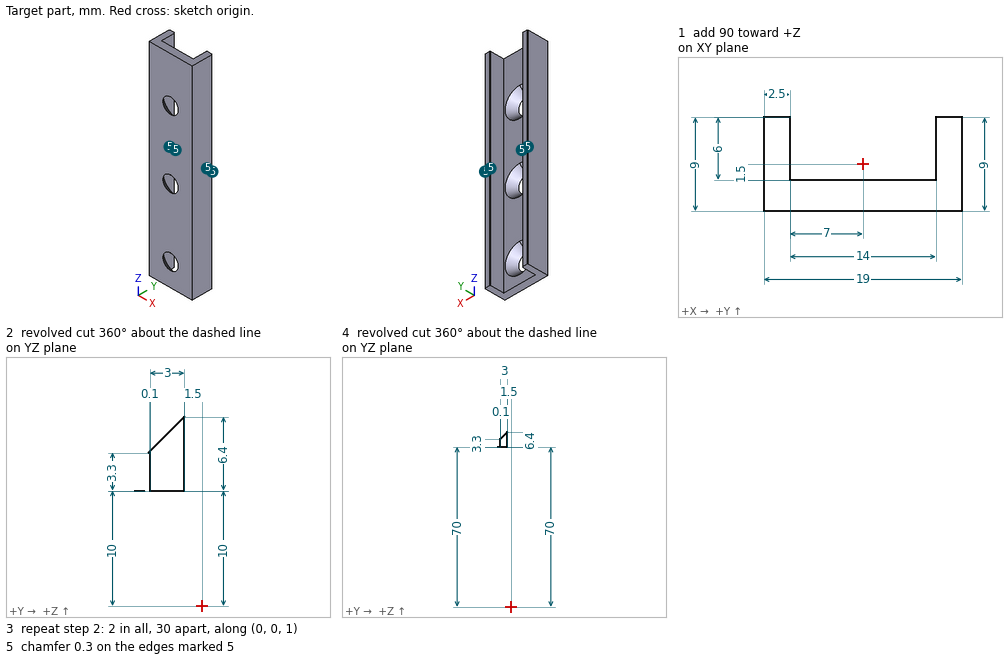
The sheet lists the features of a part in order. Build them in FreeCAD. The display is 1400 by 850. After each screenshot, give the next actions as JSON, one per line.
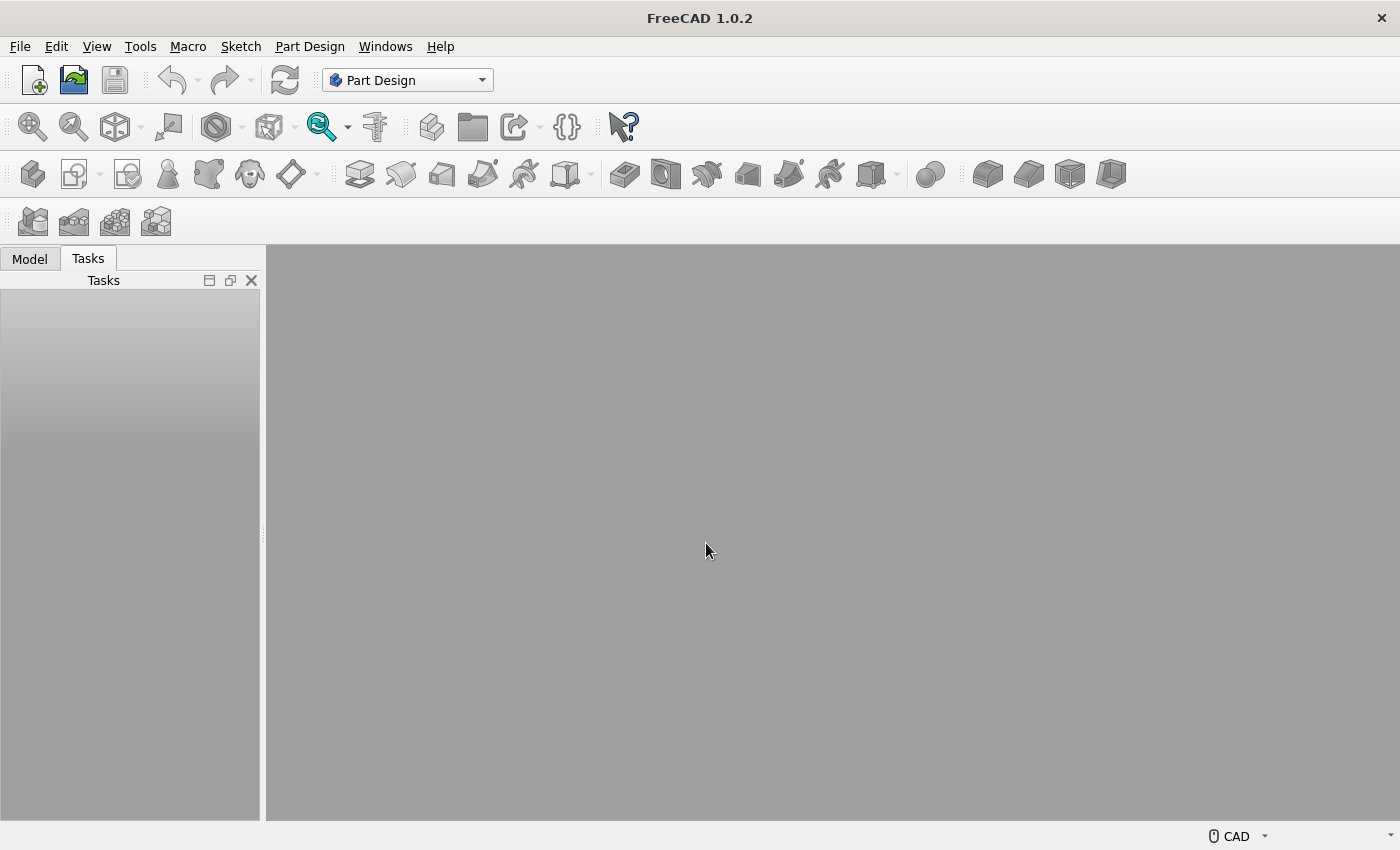
{"action": "left_click", "coordinate": [33, 80]}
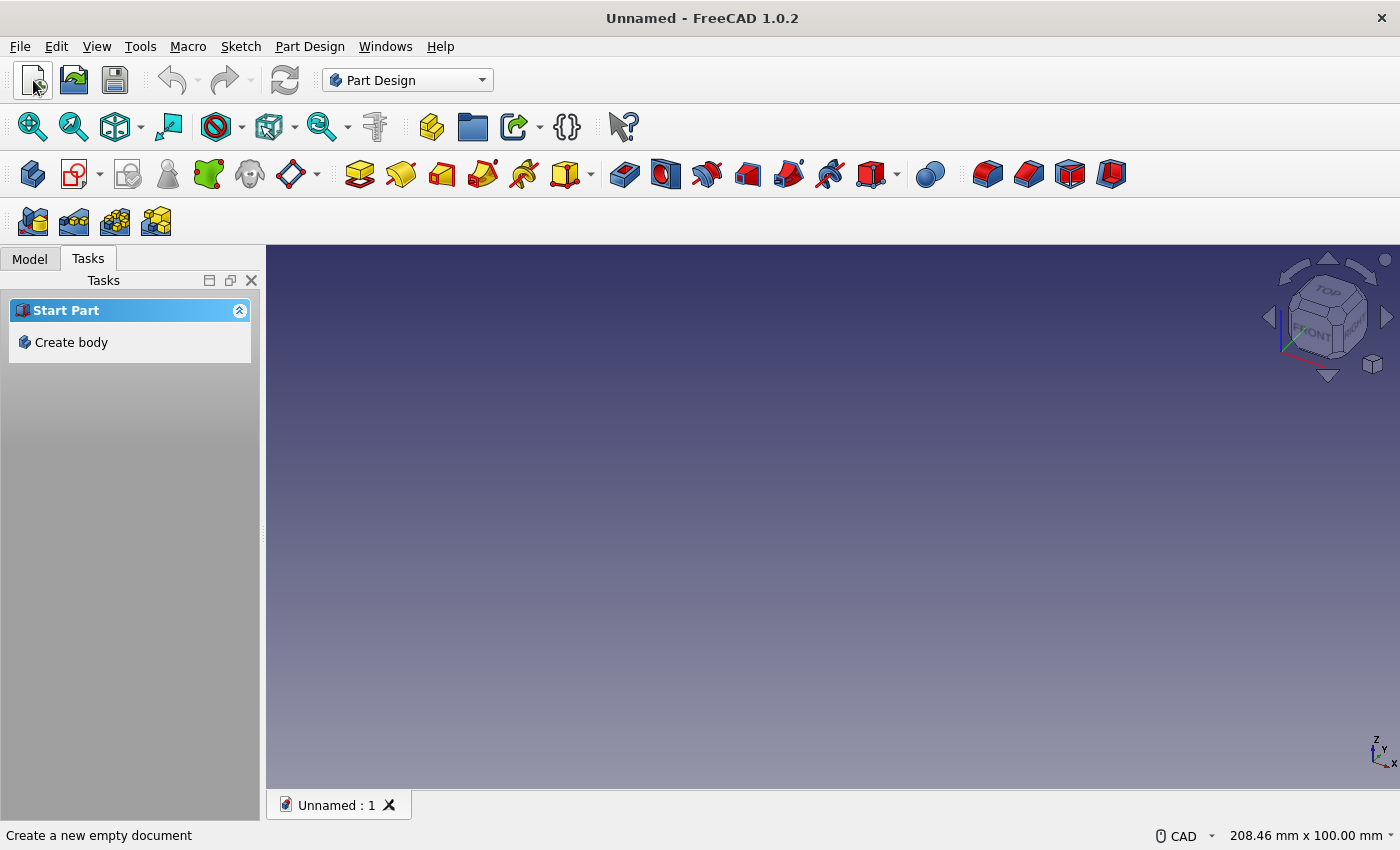
{"action": "left_click", "coordinate": [74, 174]}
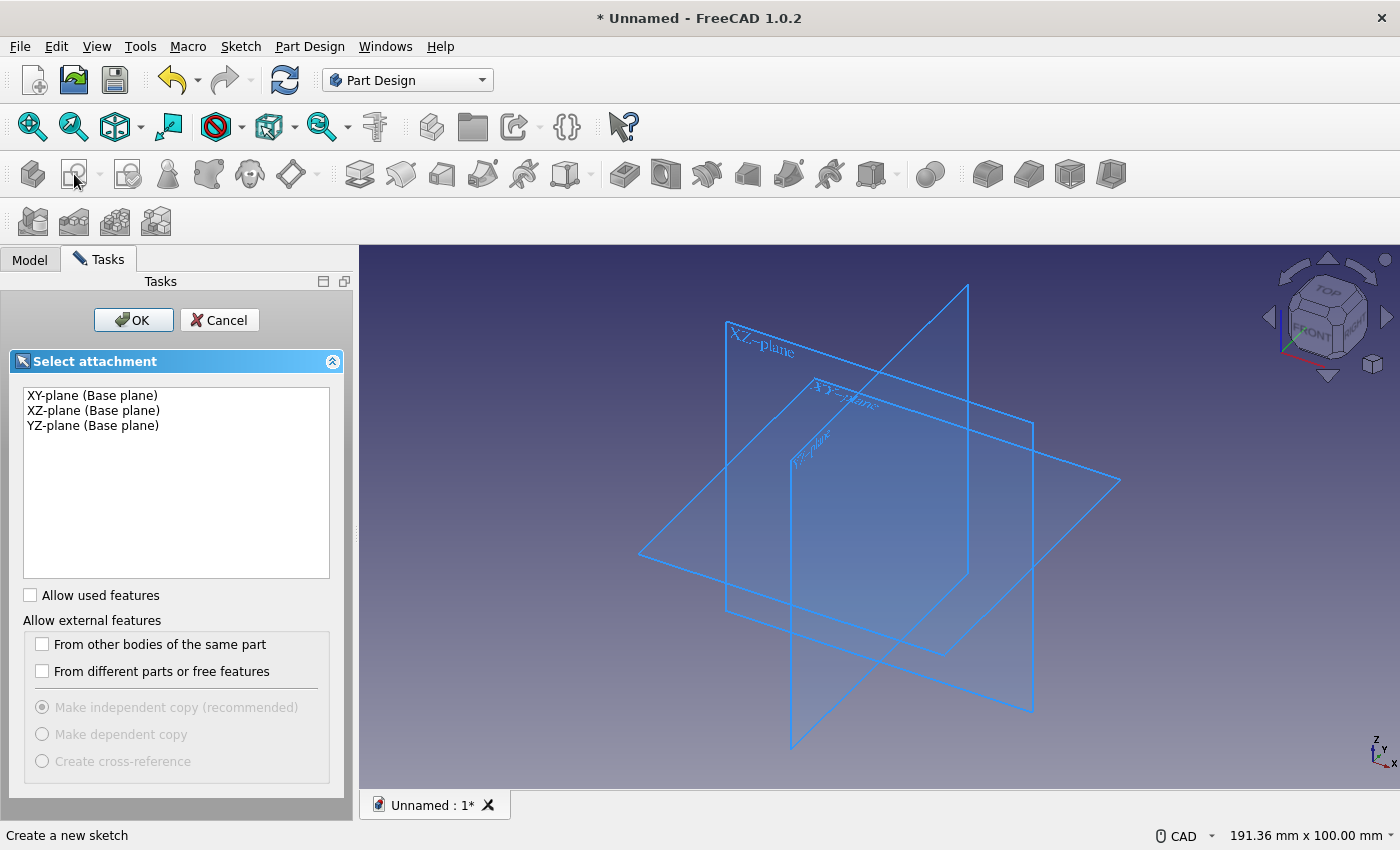
{"action": "left_click", "coordinate": [84, 396]}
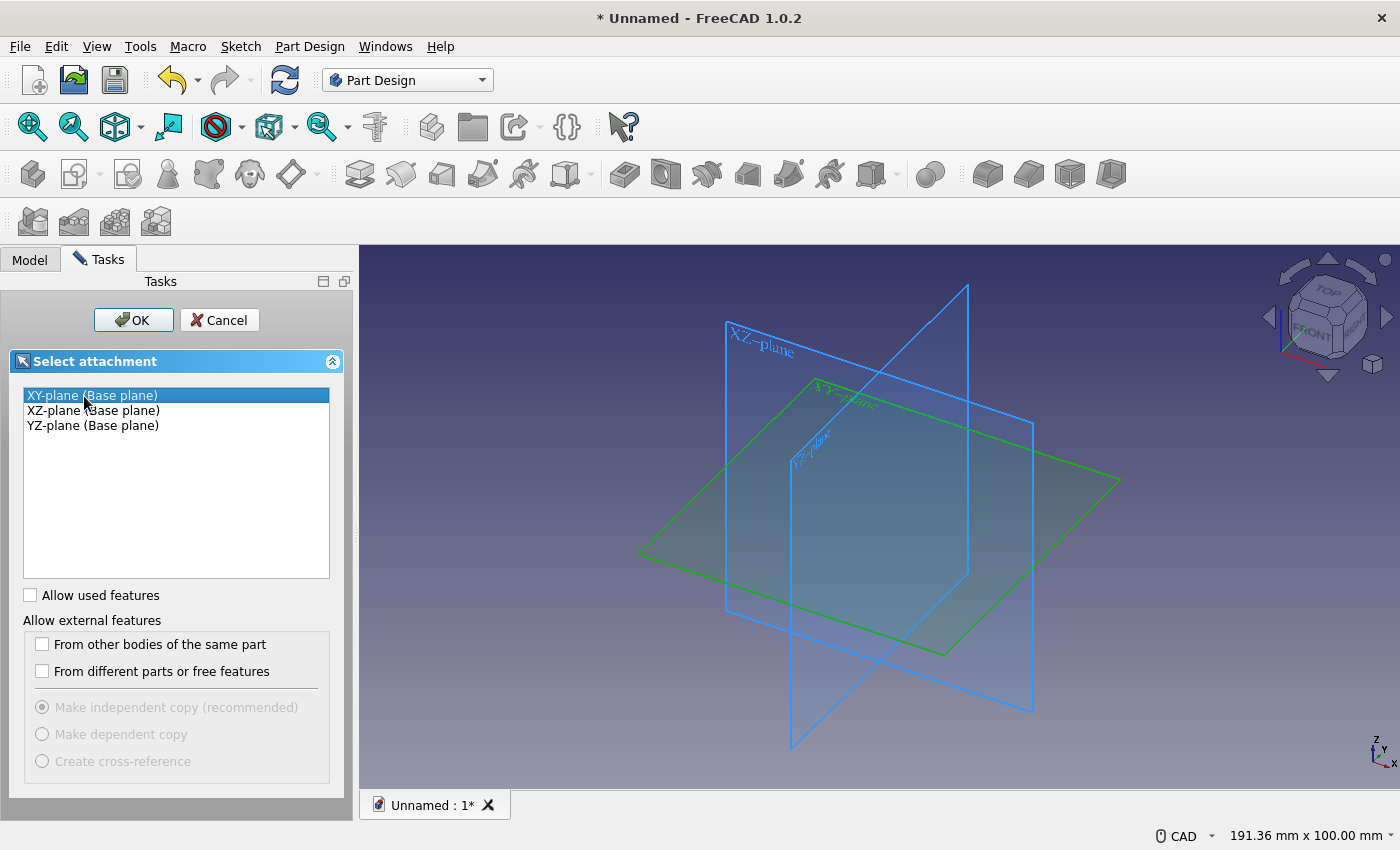
{"action": "left_click", "coordinate": [134, 320]}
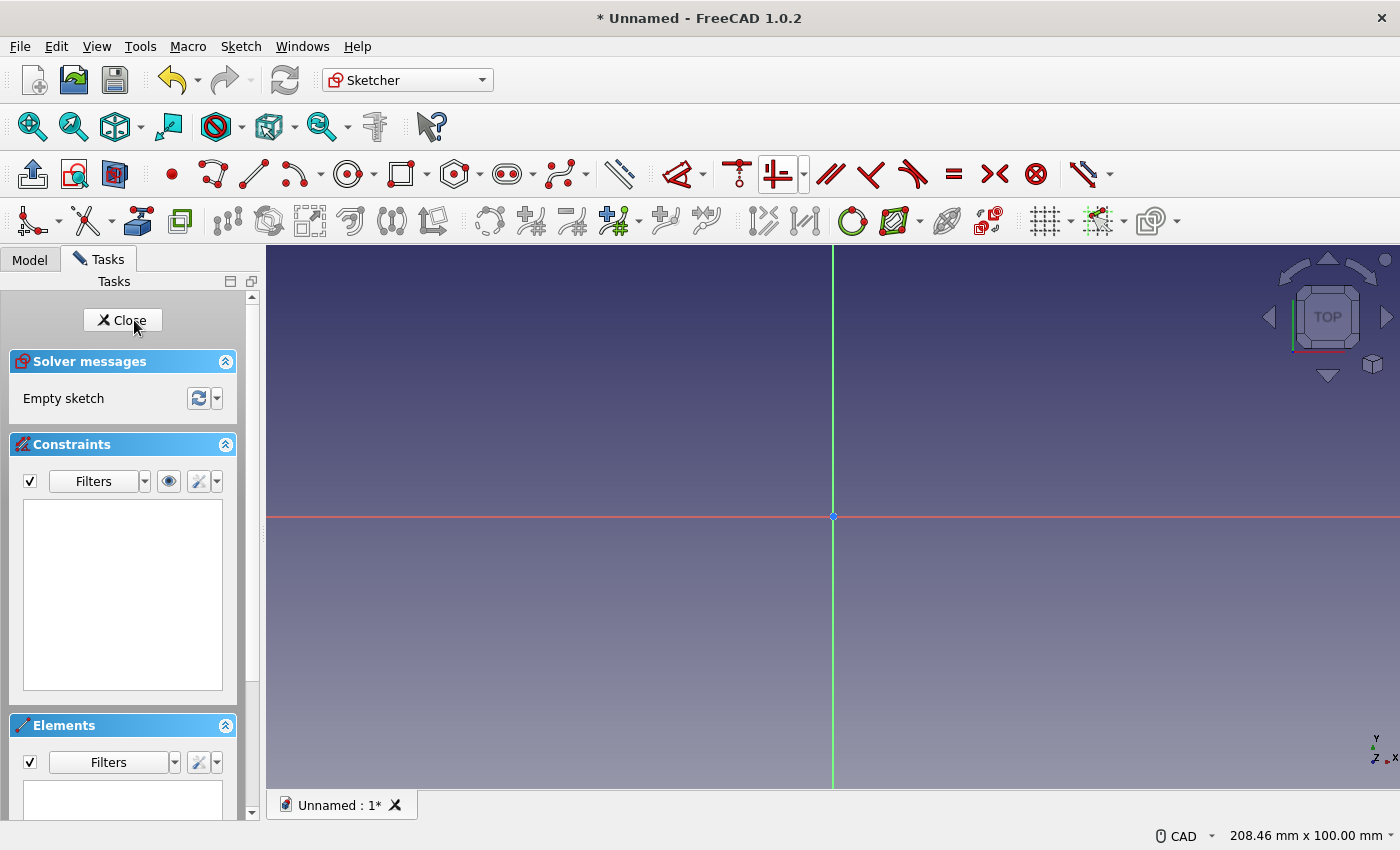
{"action": "scroll", "coordinate": [847, 517], "scroll_direction": "up", "scroll_amount": 9}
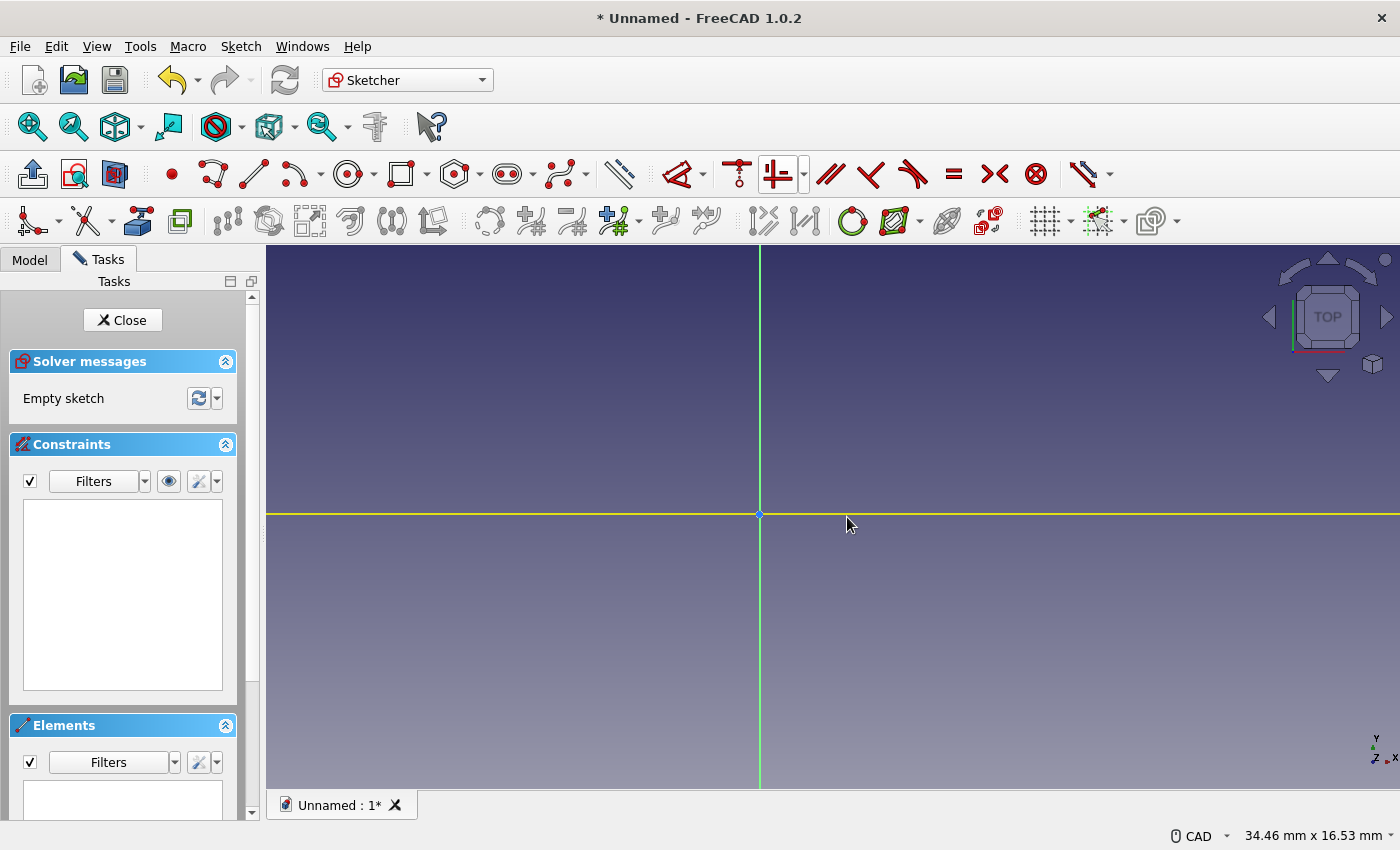
{"action": "left_click", "coordinate": [213, 174]}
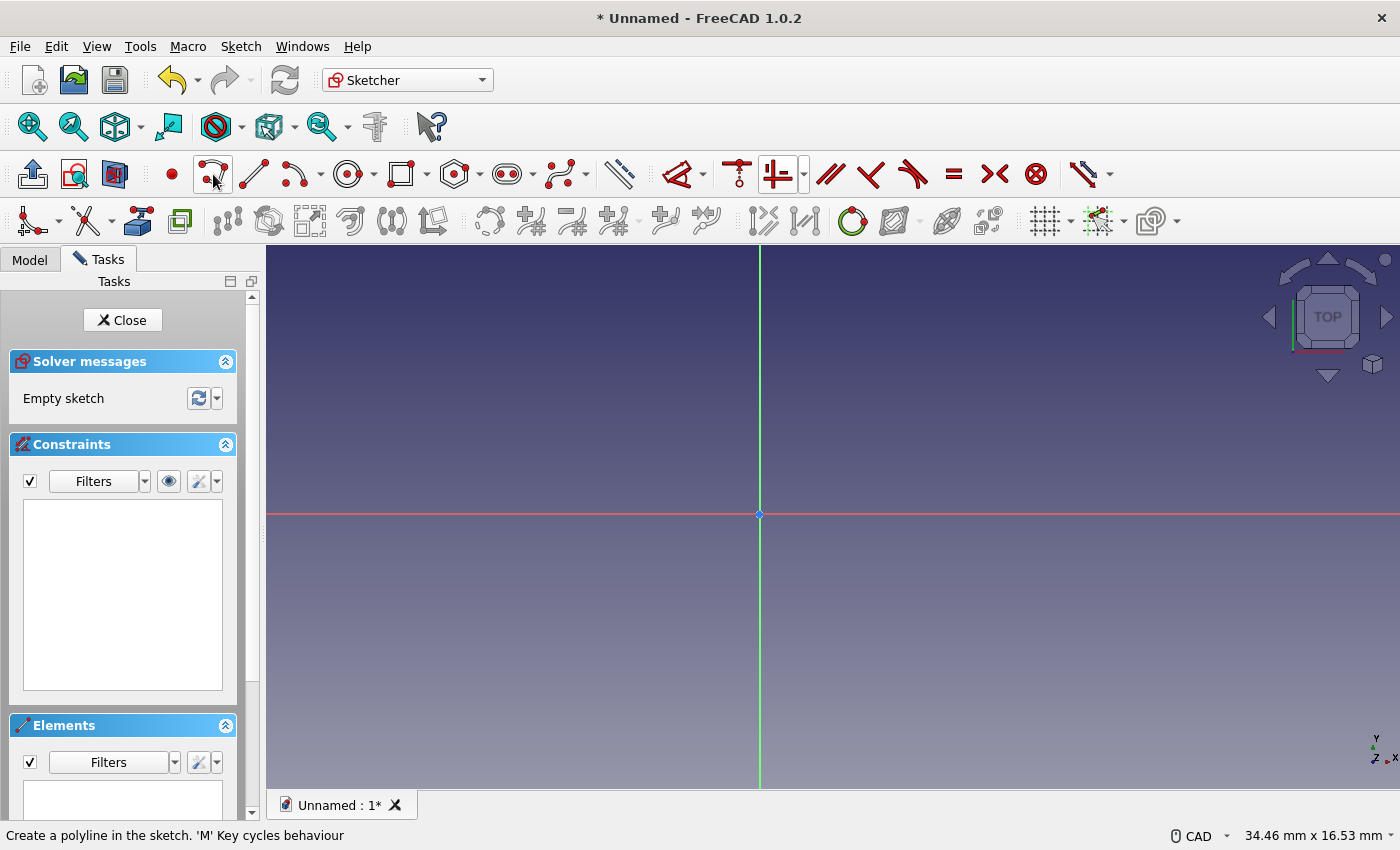
{"action": "left_click", "coordinate": [529, 564]}
{"action": "left_click", "coordinate": [529, 366]}
{"action": "left_click", "coordinate": [447, 366]}
{"action": "left_click", "coordinate": [447, 663]}
{"action": "left_click", "coordinate": [1072, 663]}
{"action": "left_click", "coordinate": [1072, 366]}
{"action": "left_click", "coordinate": [990, 366]}
{"action": "left_click", "coordinate": [990, 564]}
{"action": "left_click", "coordinate": [529, 565]}
{"action": "key", "text": "Escape"}
{"action": "key", "text": "Escape"}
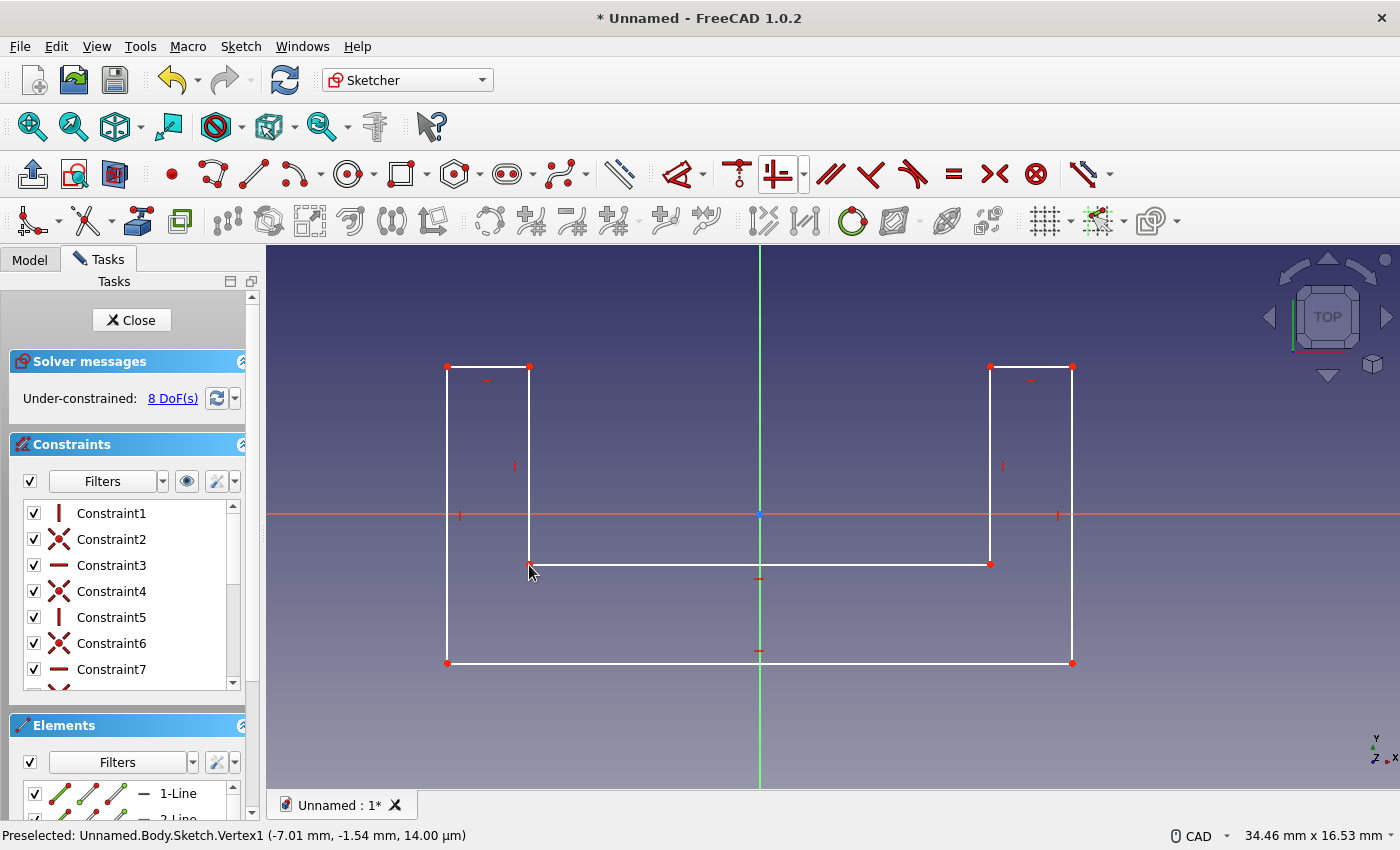
{"action": "left_click", "coordinate": [676, 174]}